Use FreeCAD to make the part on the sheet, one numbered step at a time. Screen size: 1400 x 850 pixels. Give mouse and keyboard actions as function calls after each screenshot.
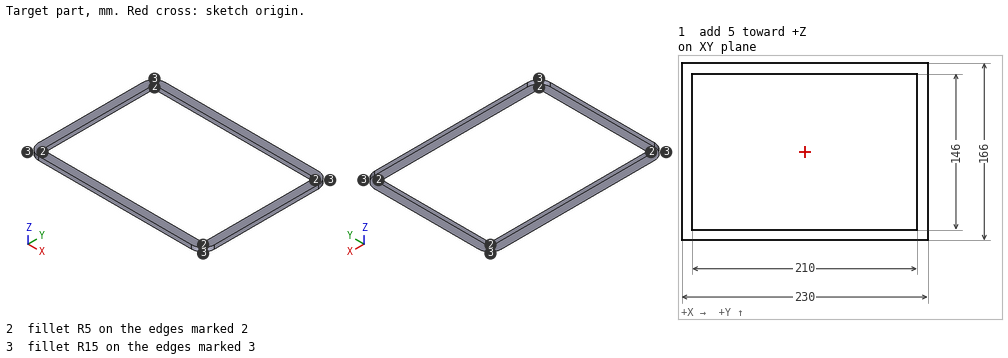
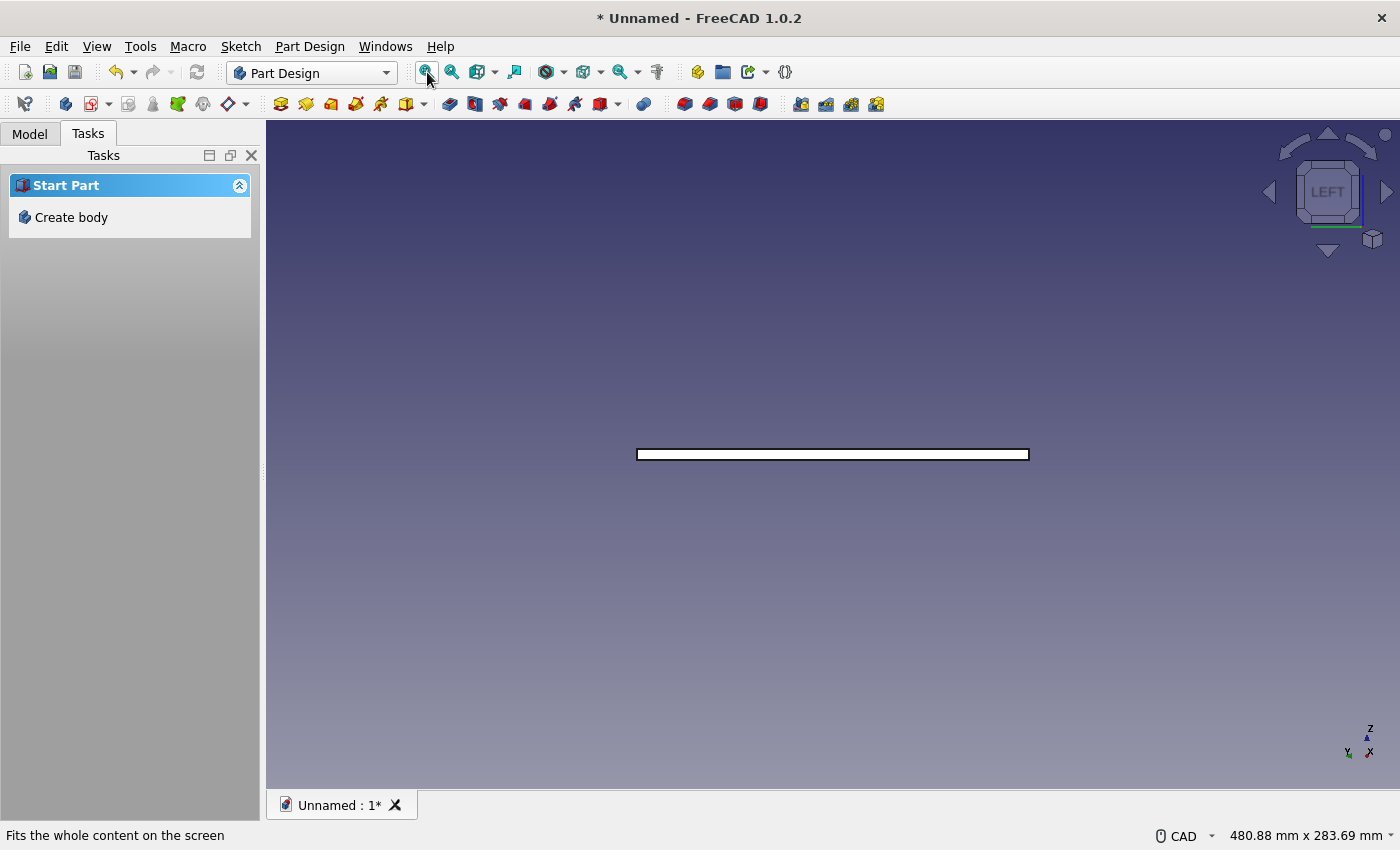
scroll(661, 453, up, 7)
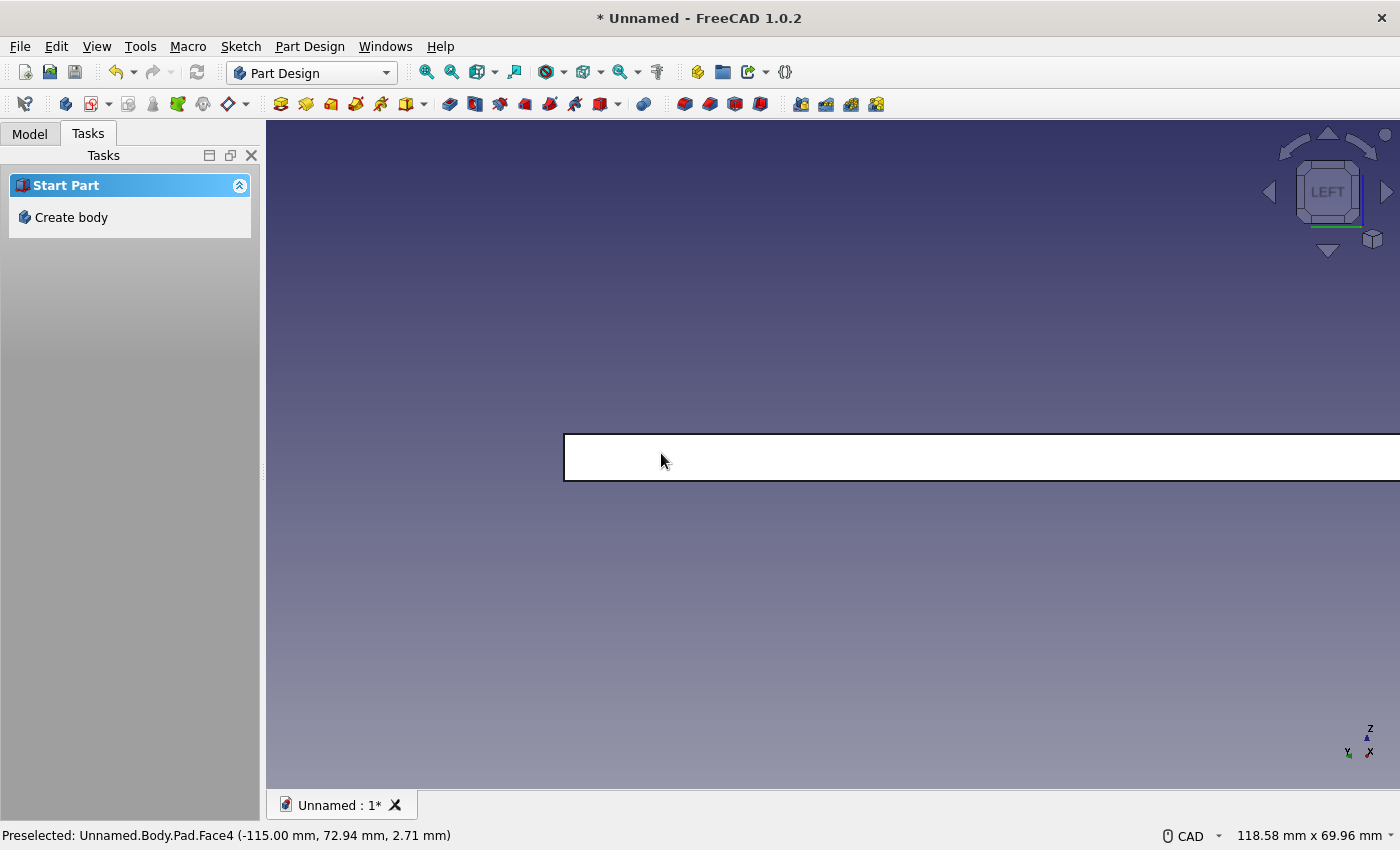
key(v)
key(f)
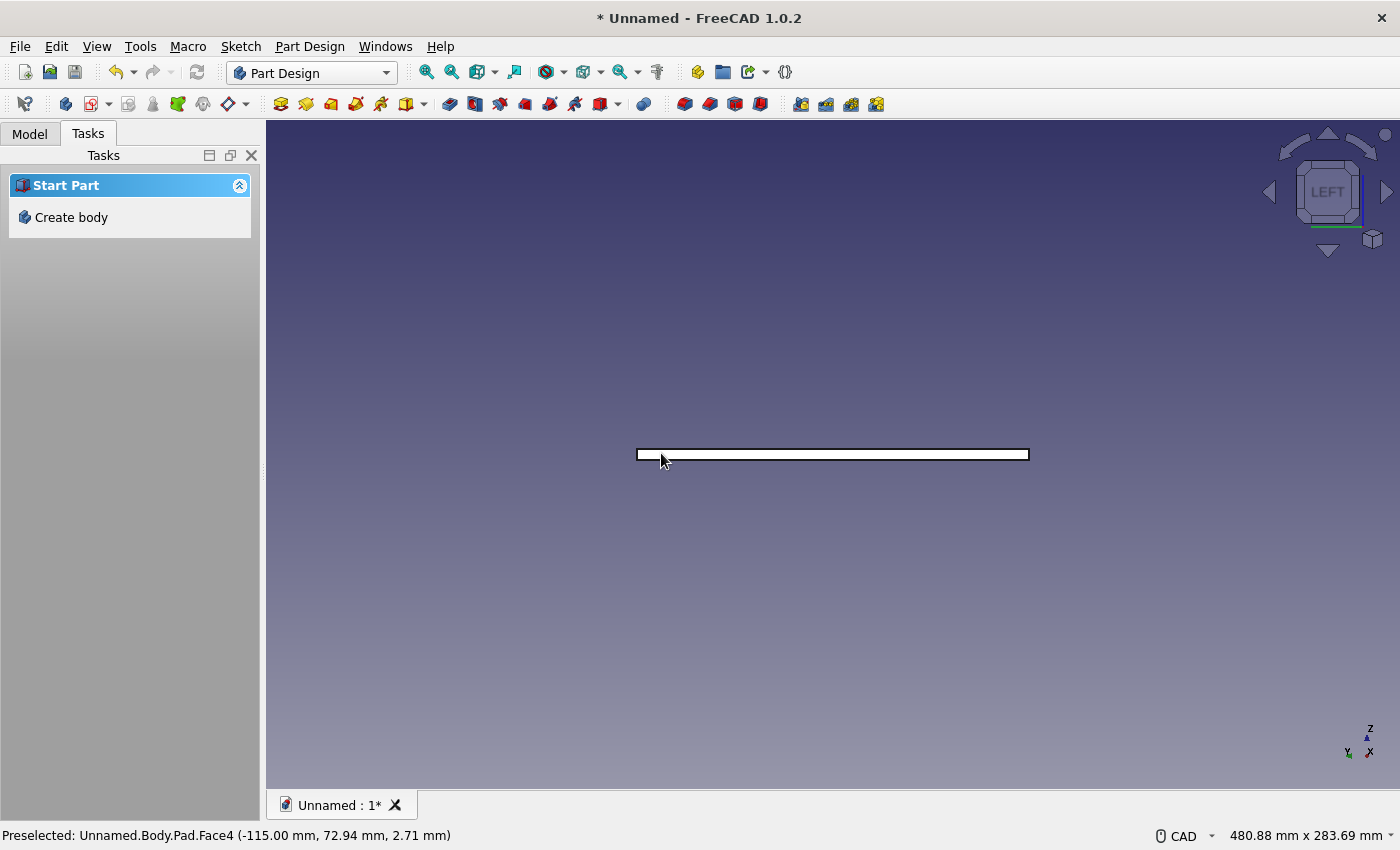
key(v)
key(3)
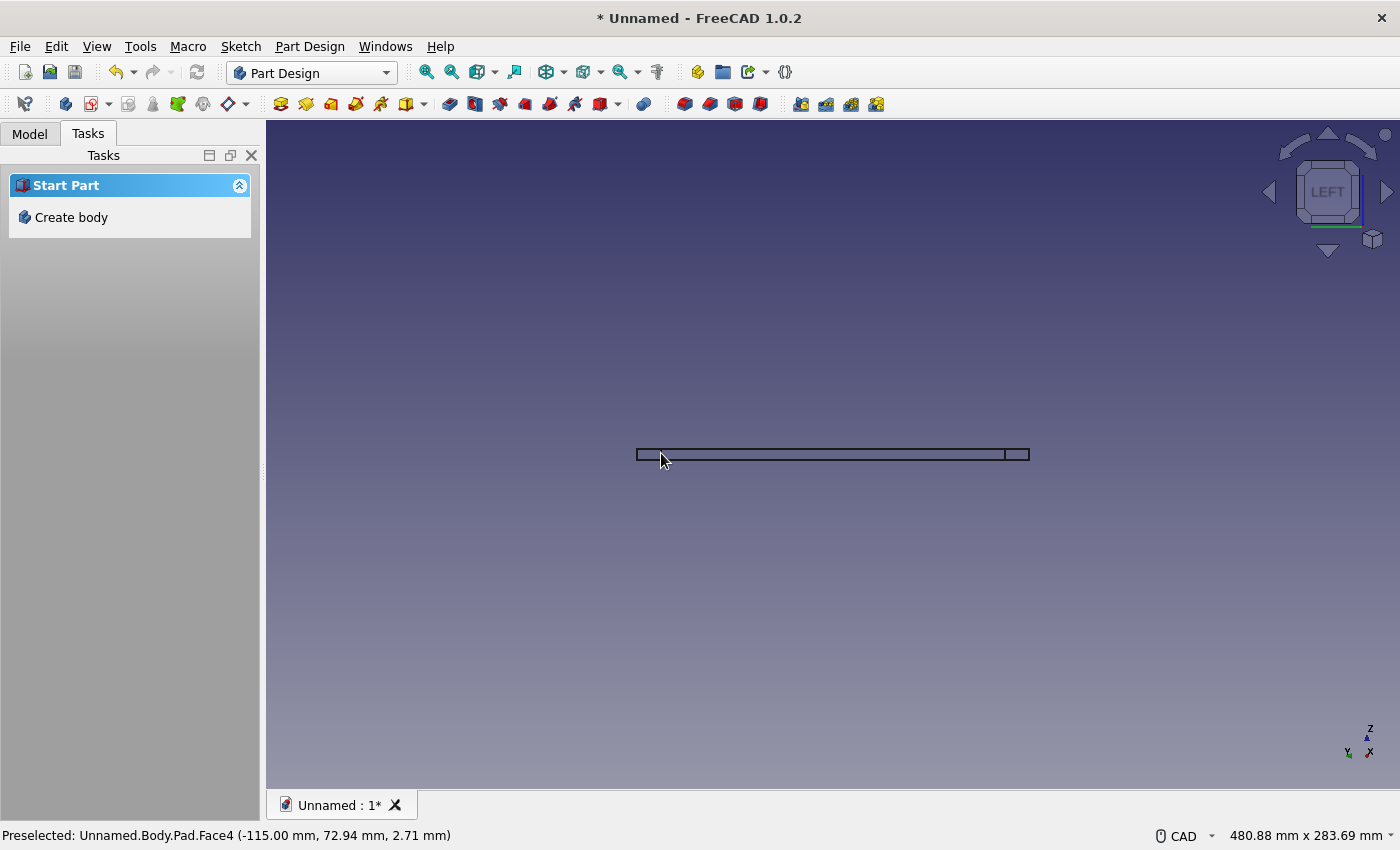
key(0)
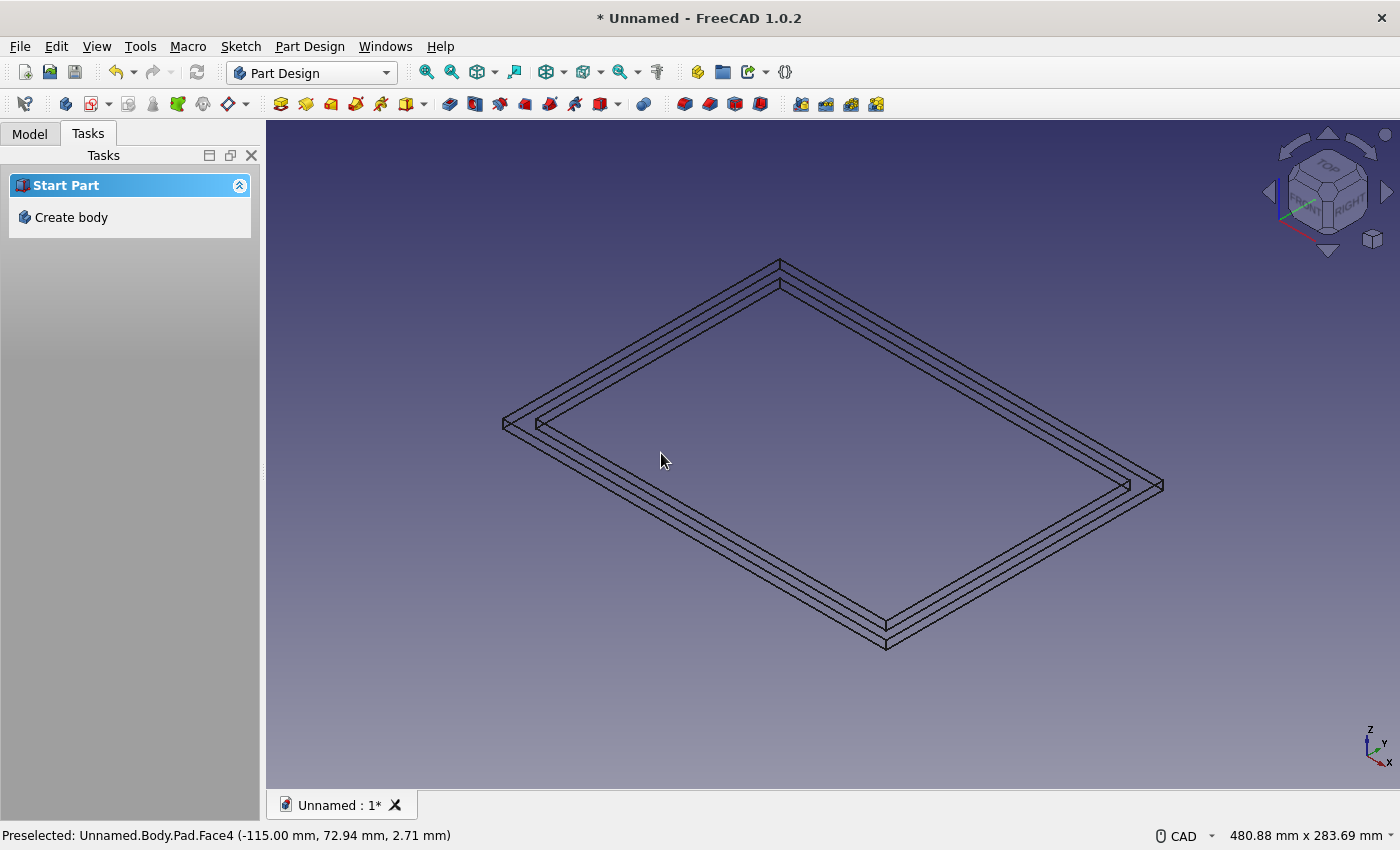
click(780, 285)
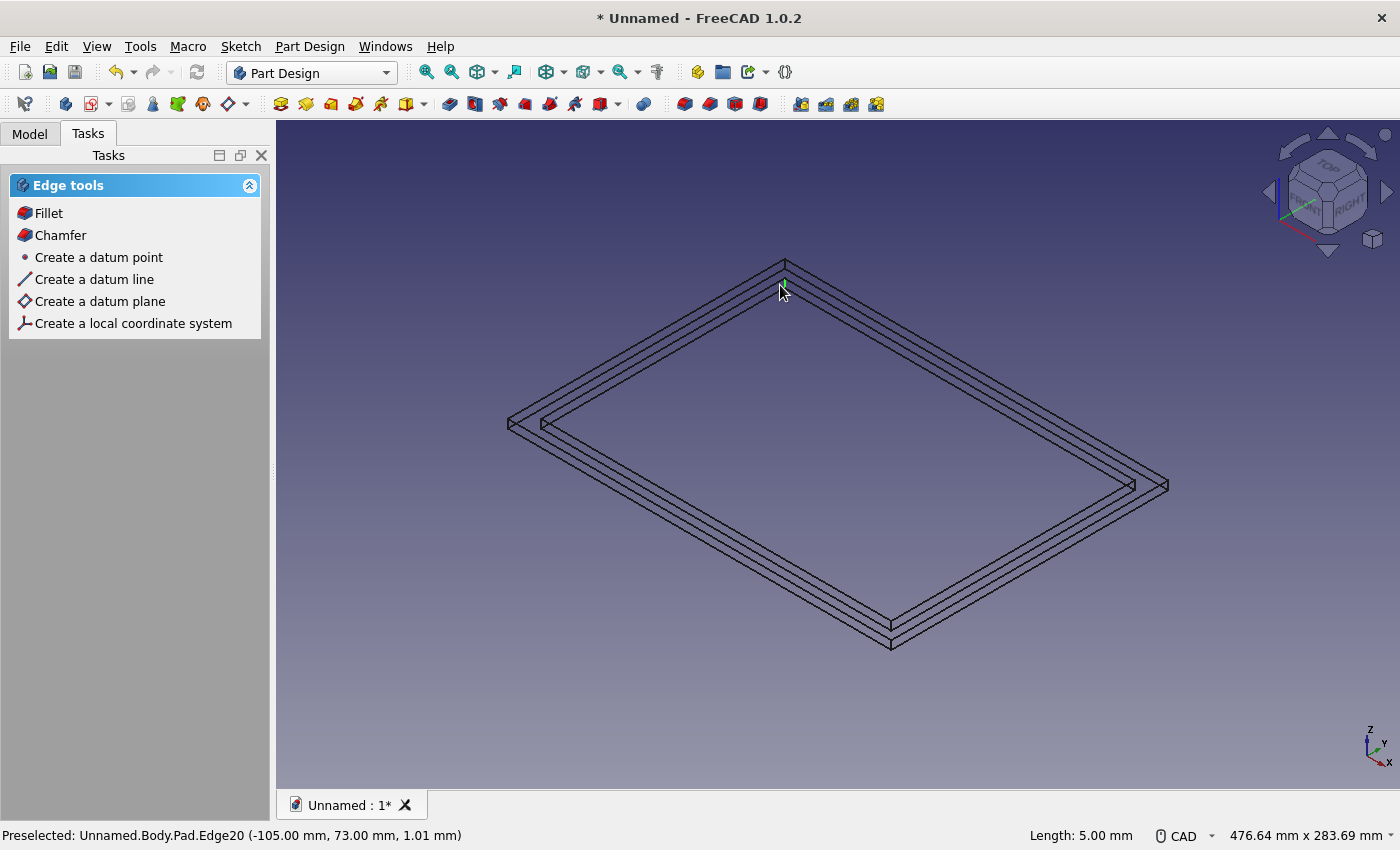
click(541, 426, ctrl)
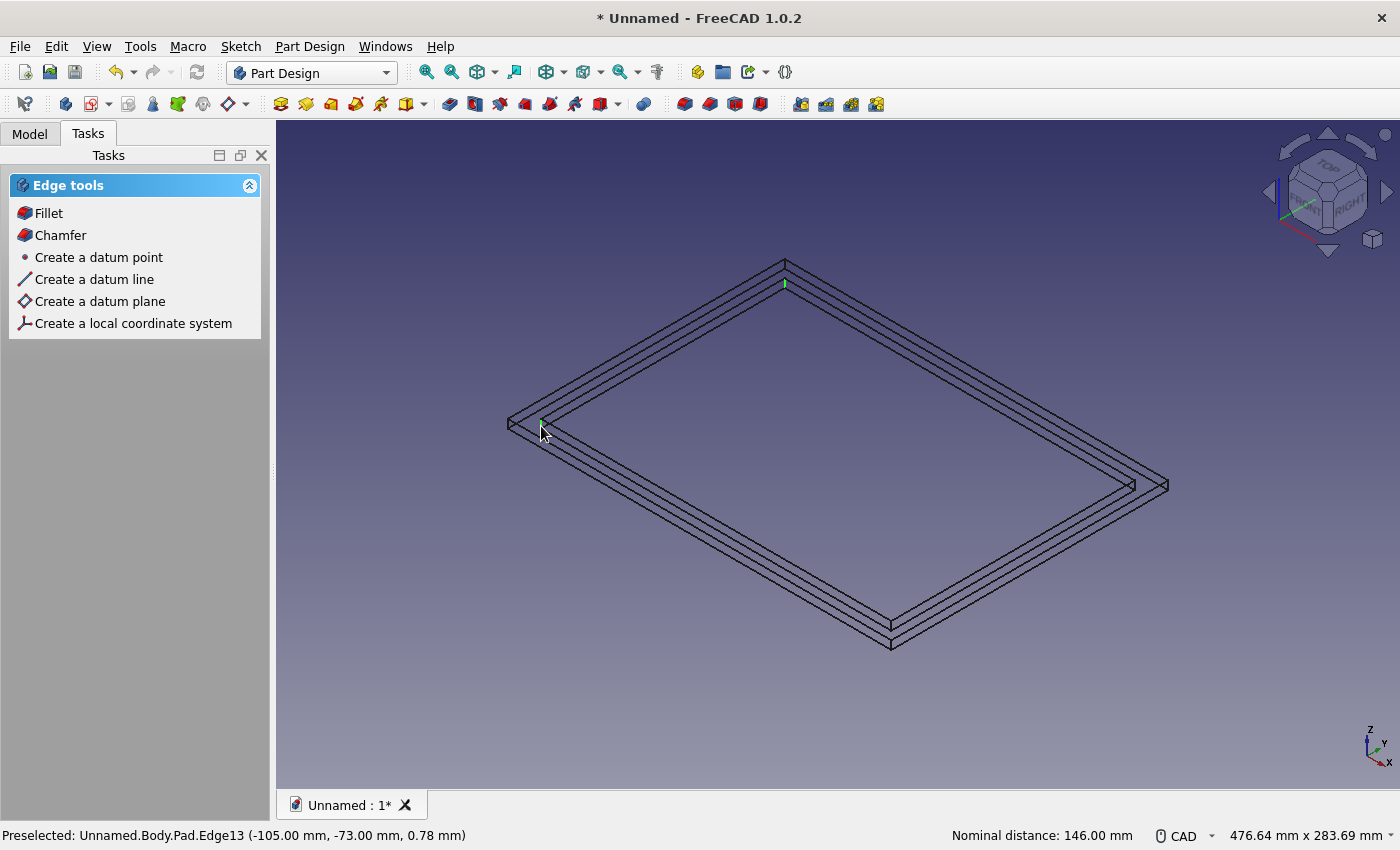
click(891, 627, ctrl)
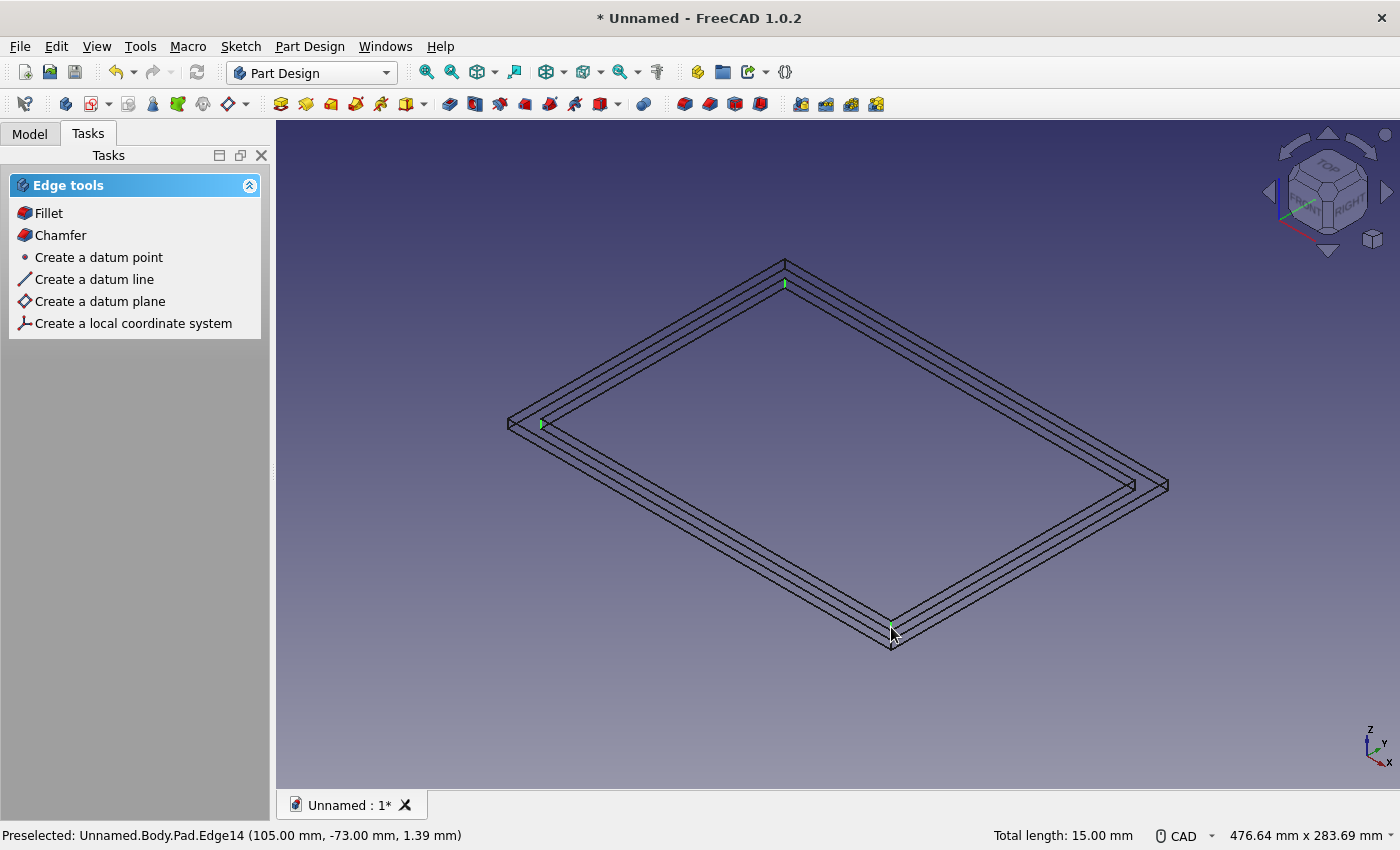
click(1135, 487, ctrl)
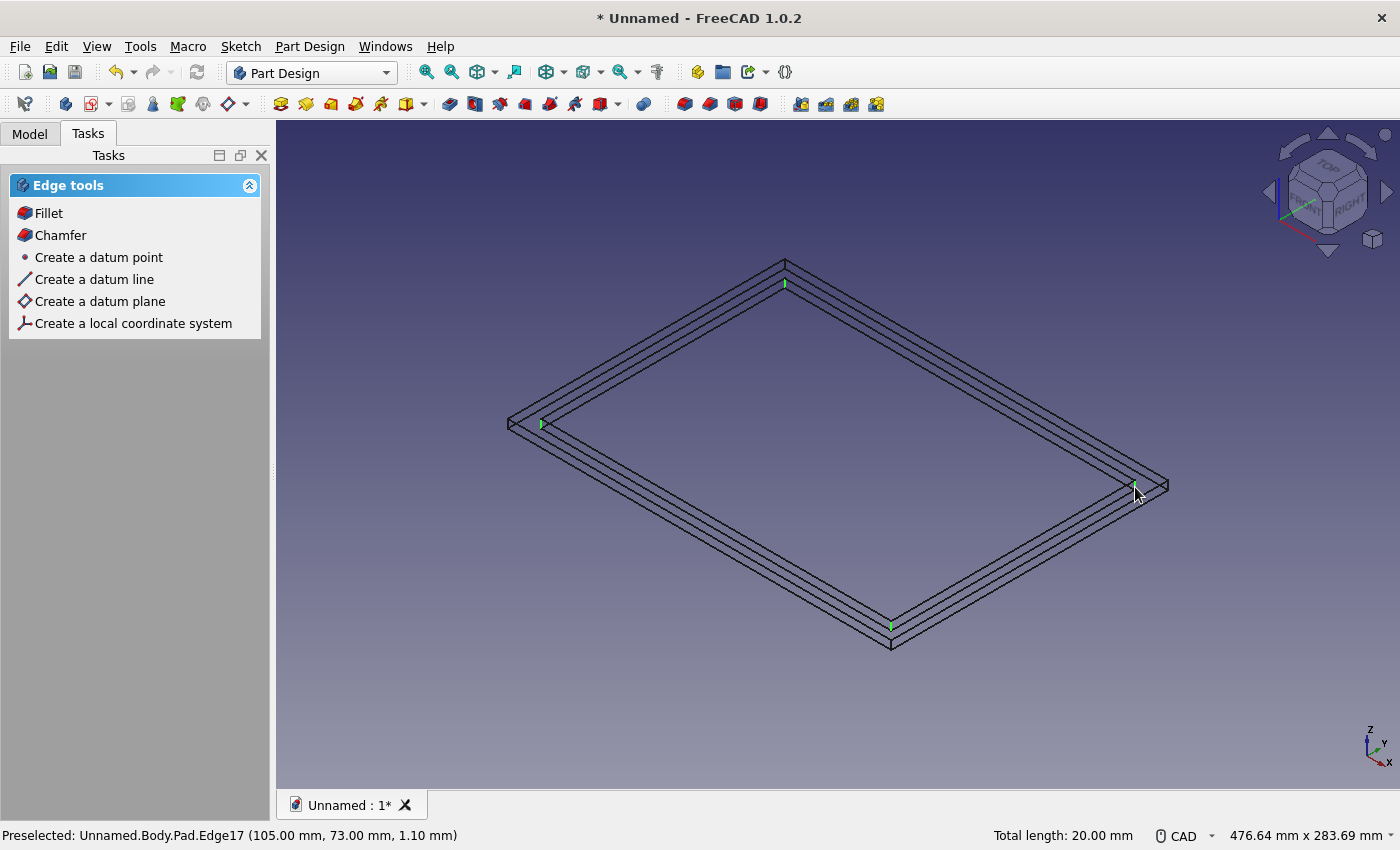
key(v)
key(1)